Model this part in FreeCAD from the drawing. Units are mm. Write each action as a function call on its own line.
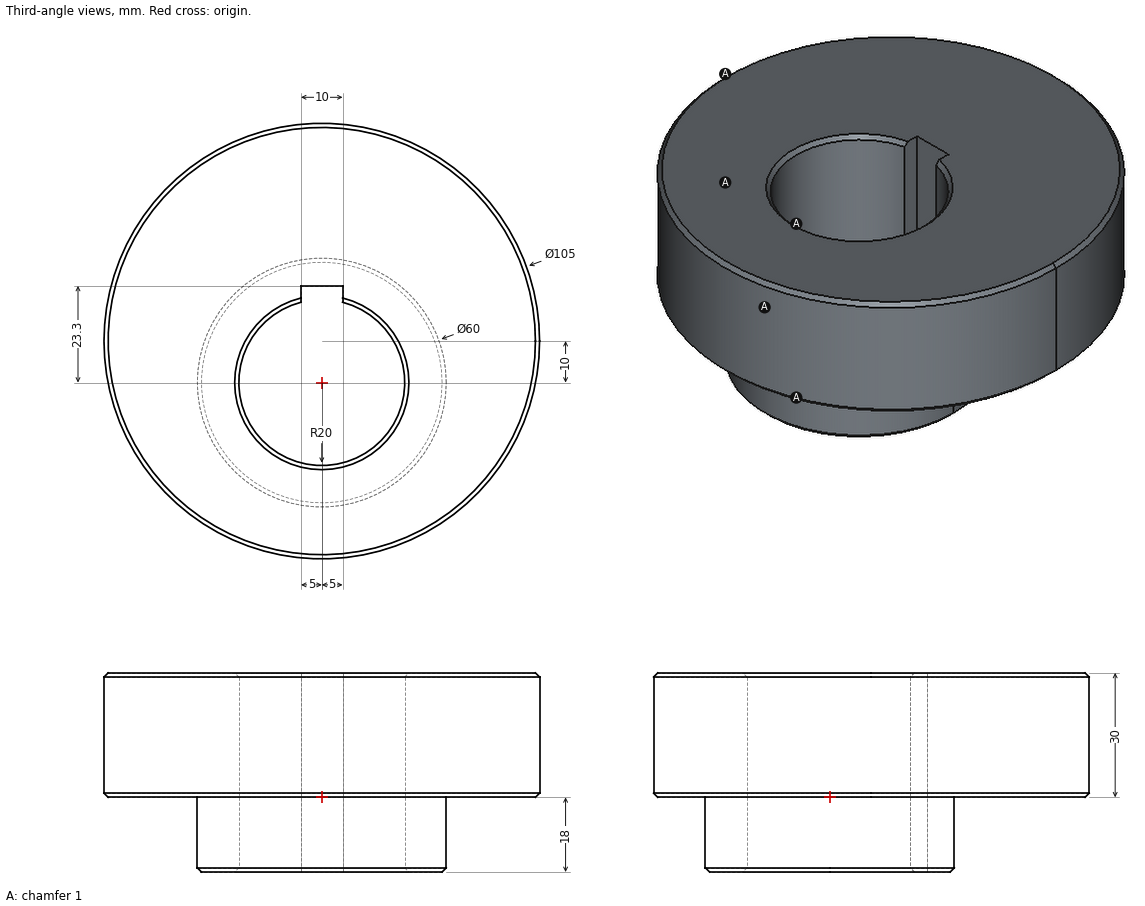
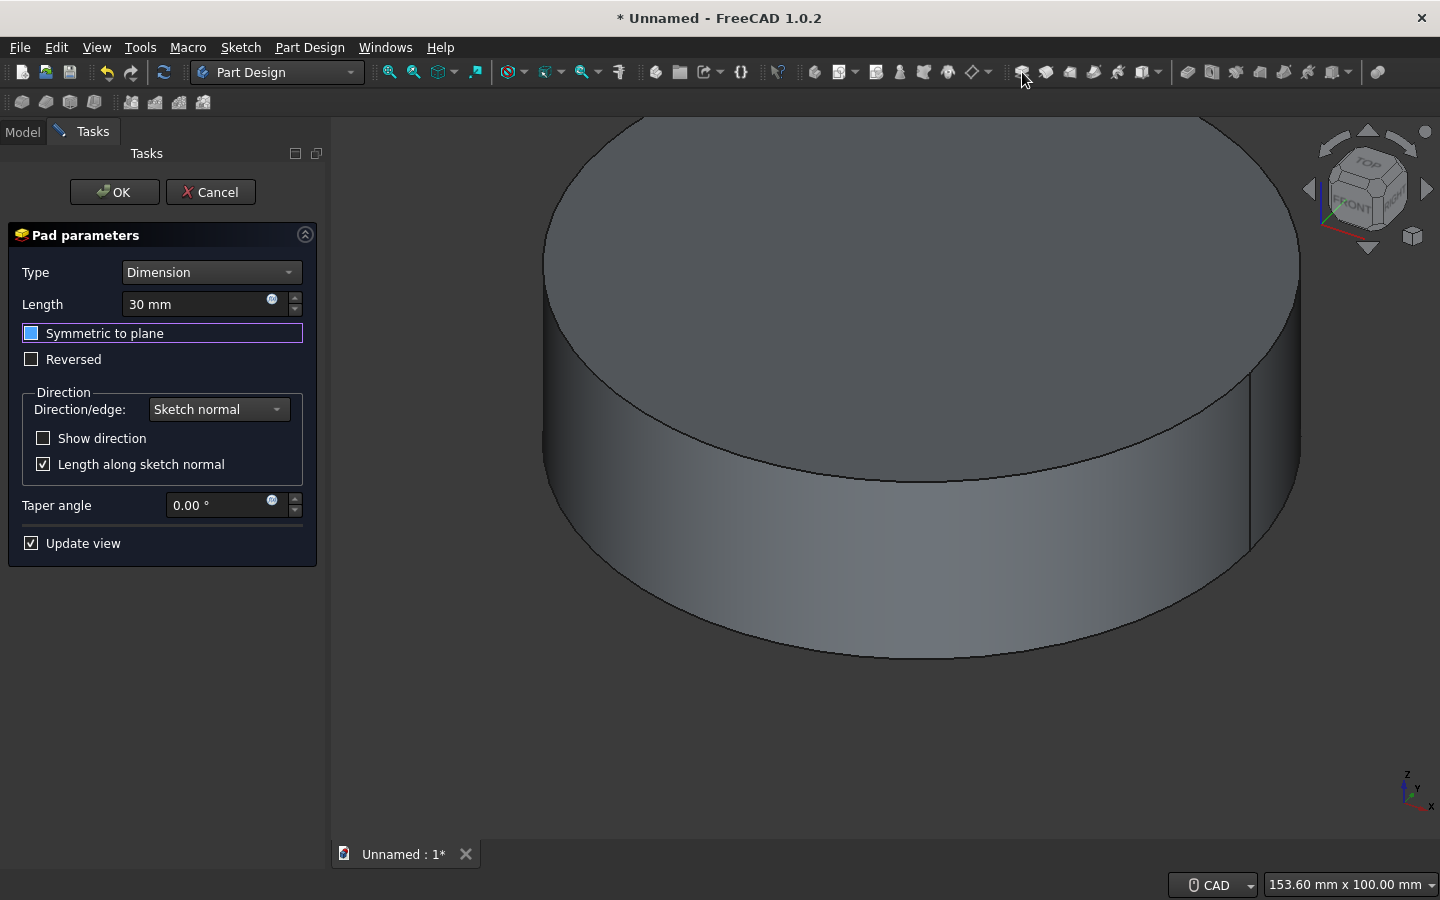
click(115, 192)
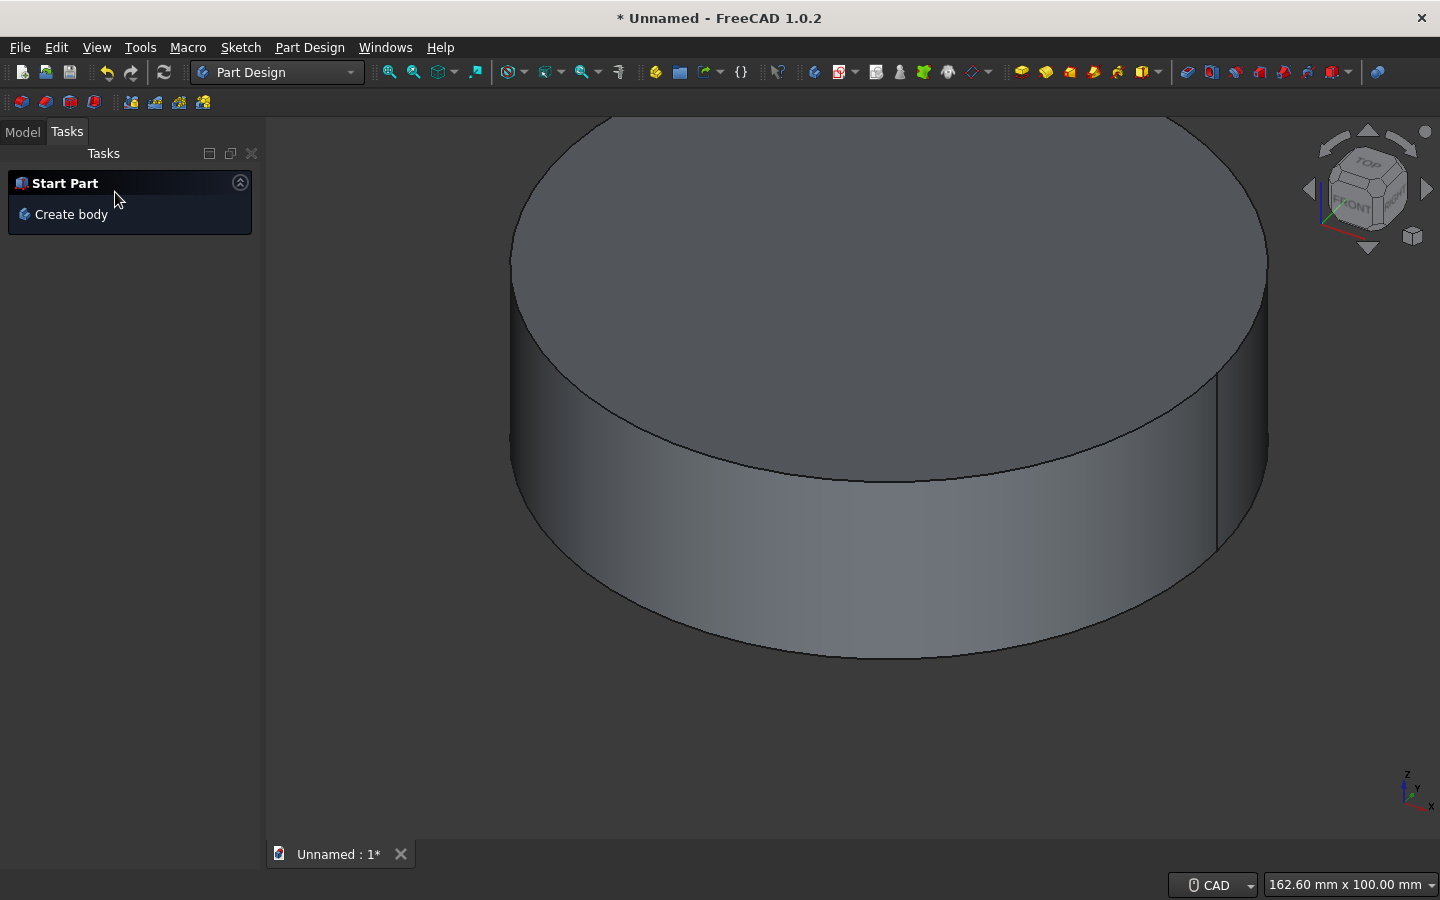
click(390, 72)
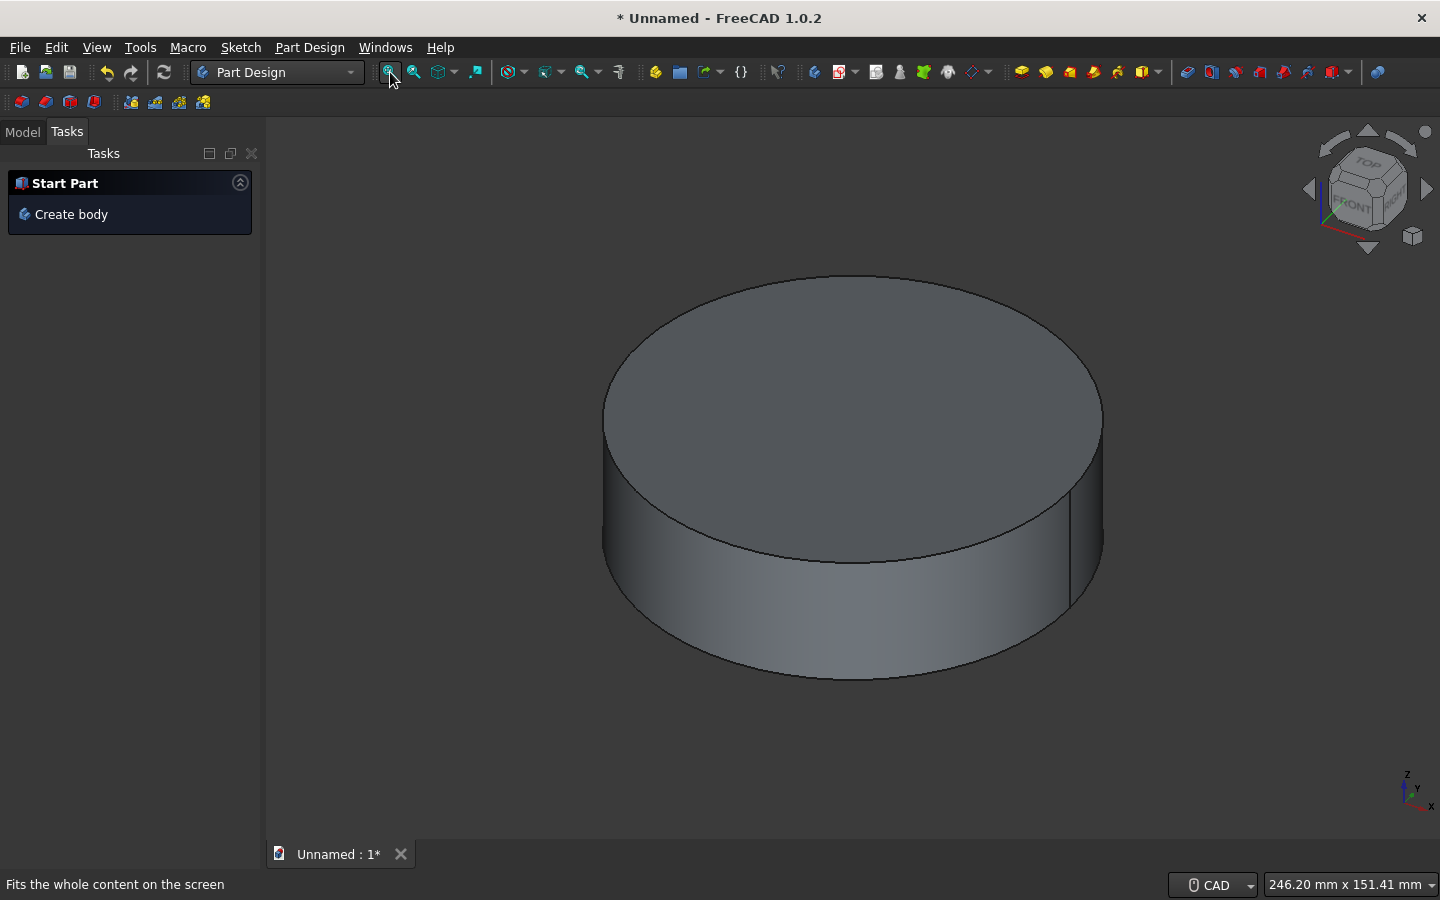
key(5)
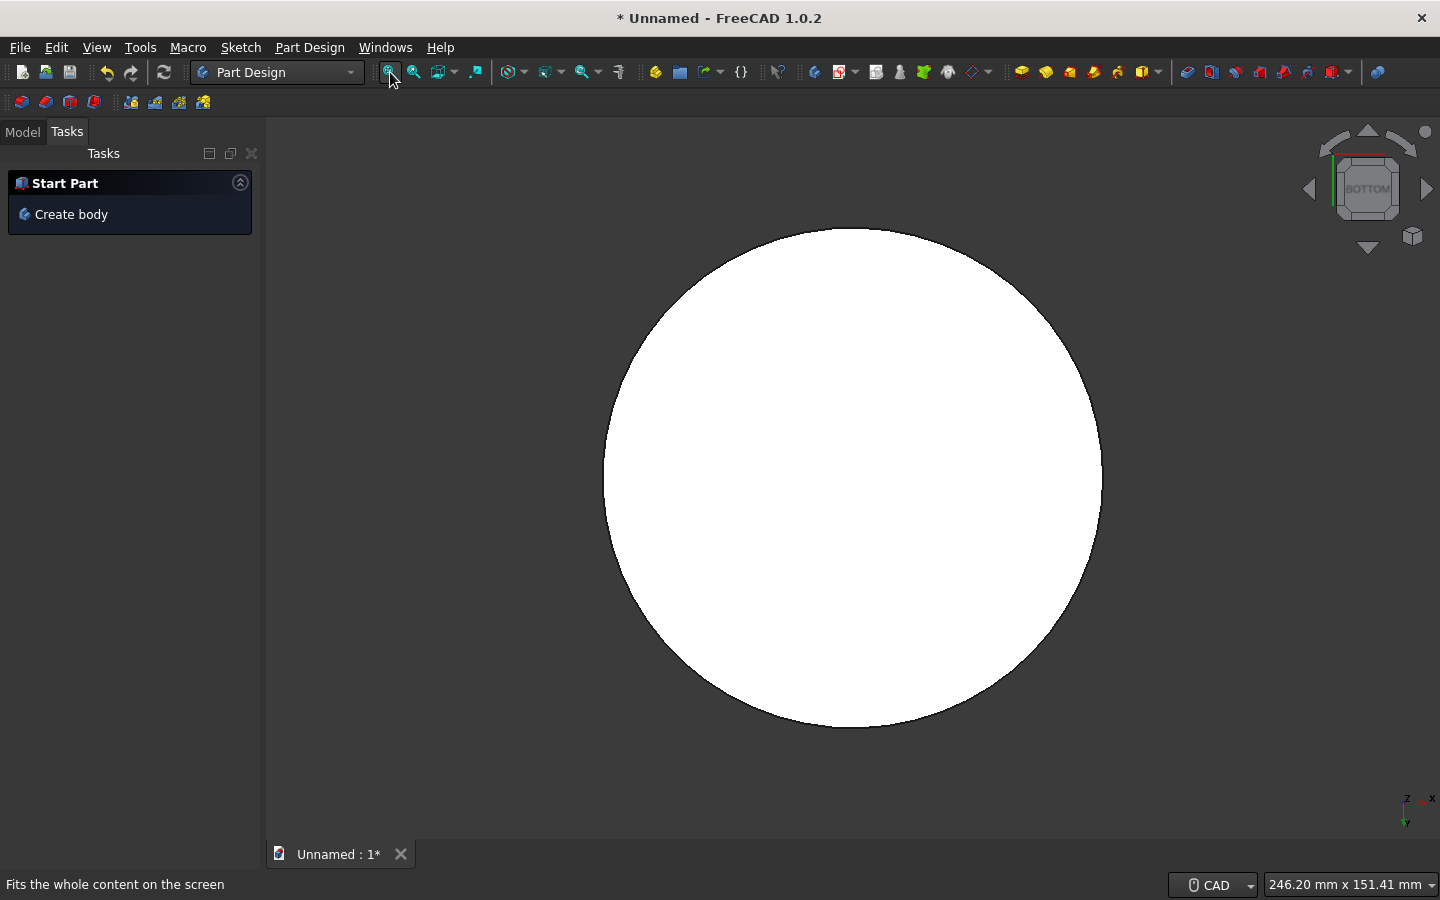
click(853, 477)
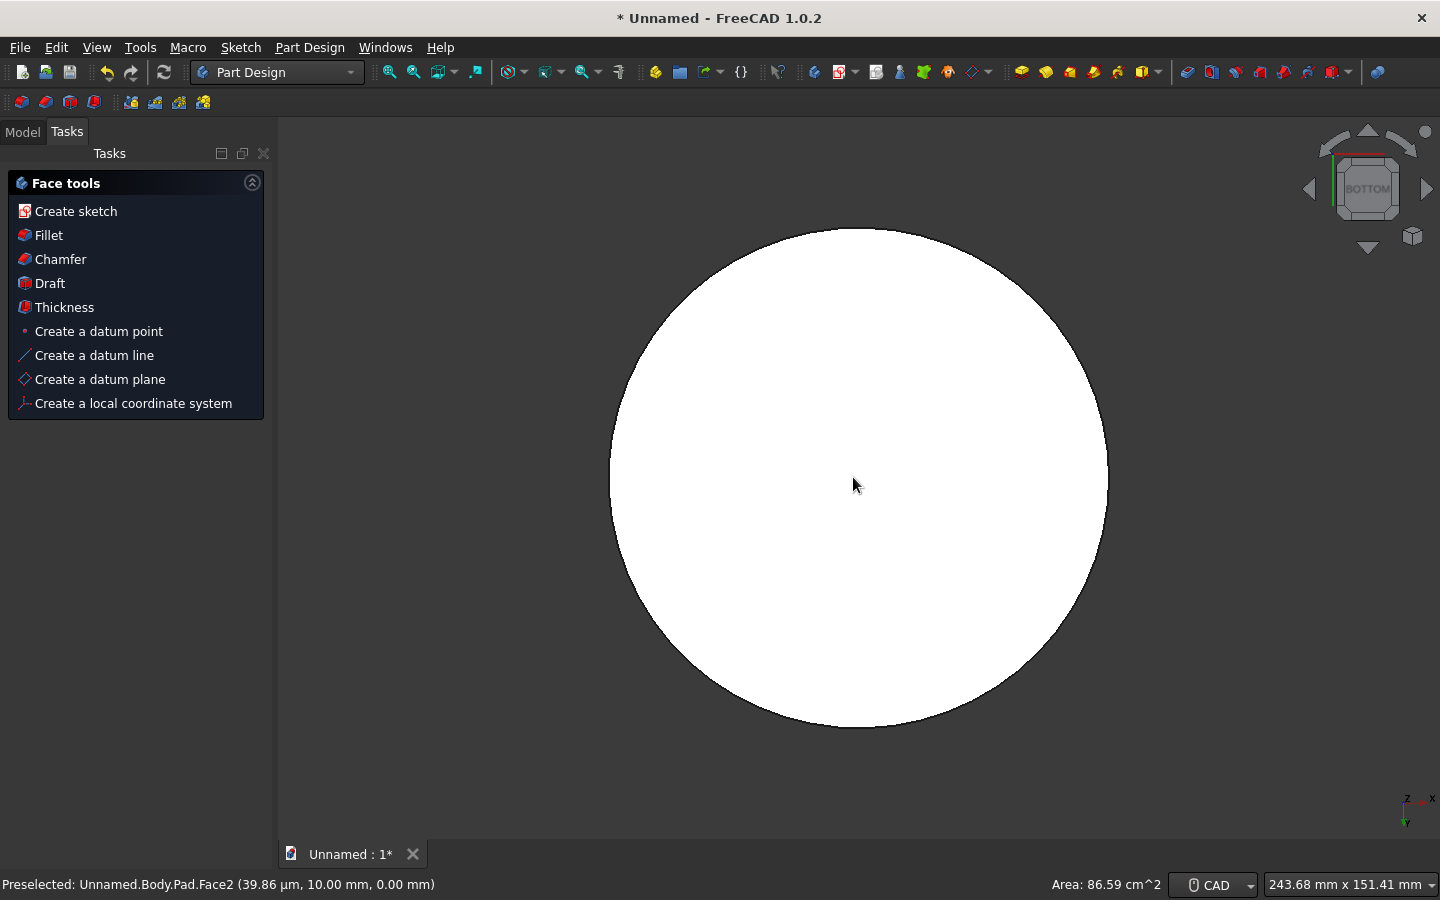
click(840, 72)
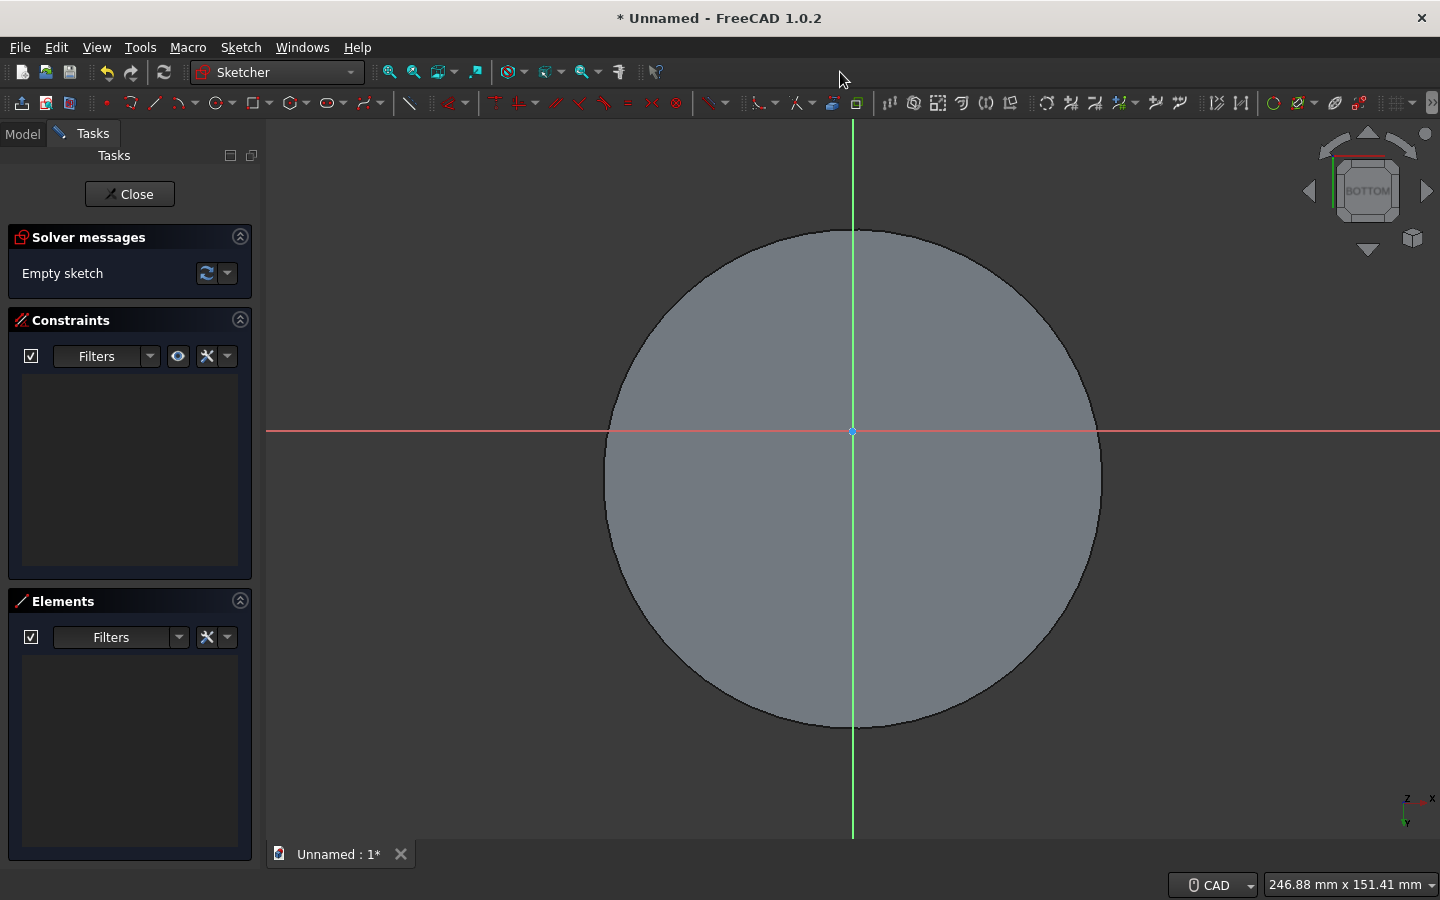
scroll(992, 335, up, 2)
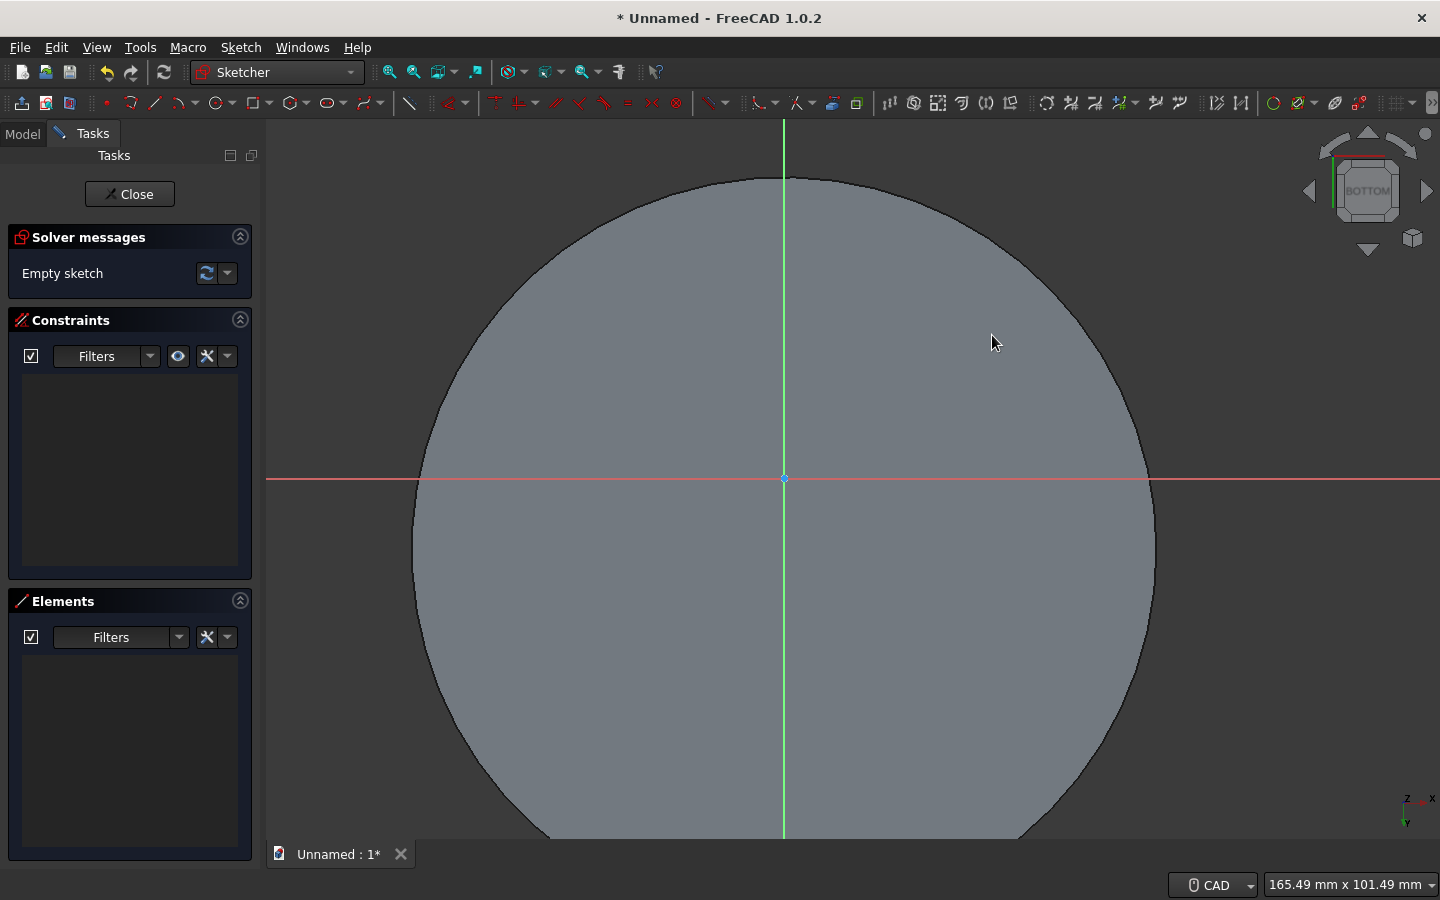
key(g)
key(m)